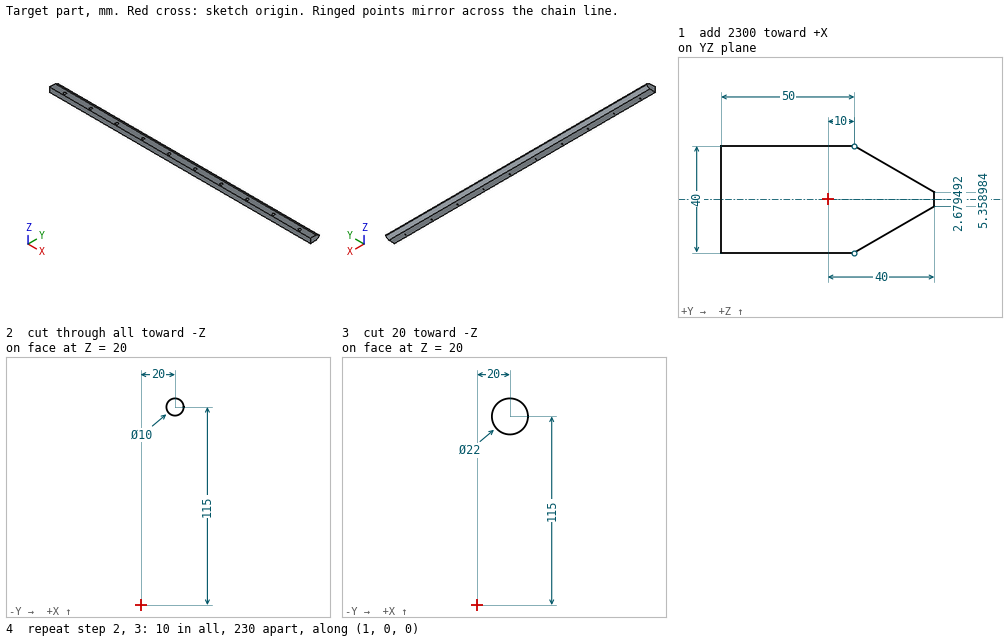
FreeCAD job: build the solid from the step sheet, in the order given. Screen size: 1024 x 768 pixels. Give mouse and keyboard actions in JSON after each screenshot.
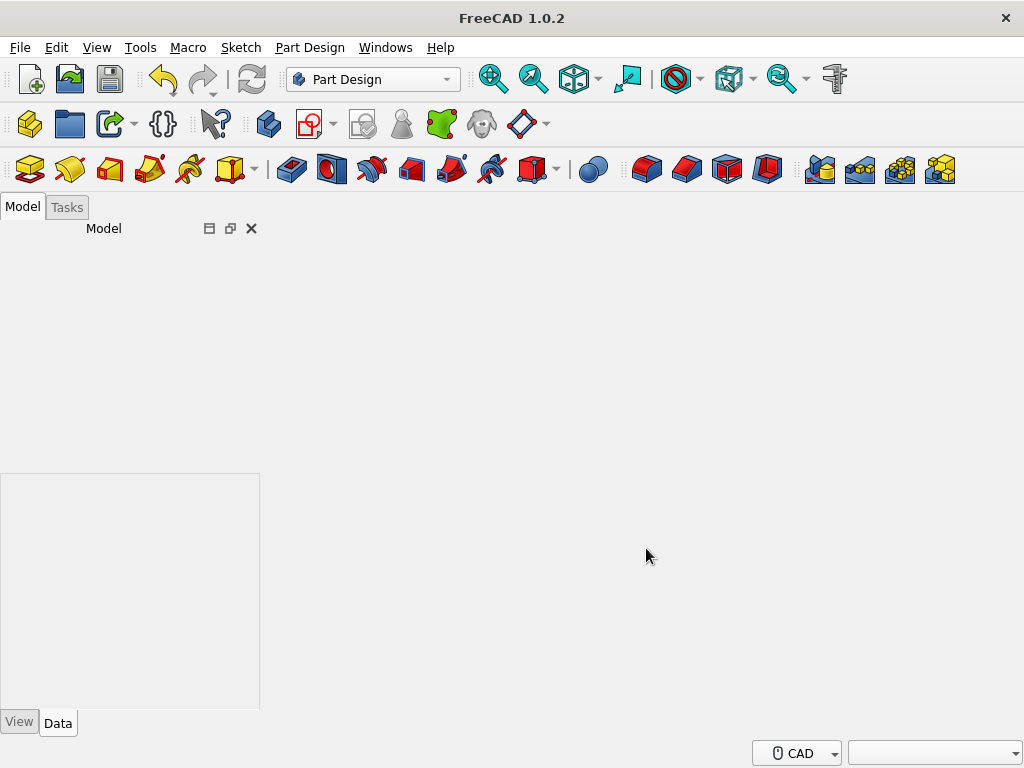
{"action": "key", "text": "ctrl+n"}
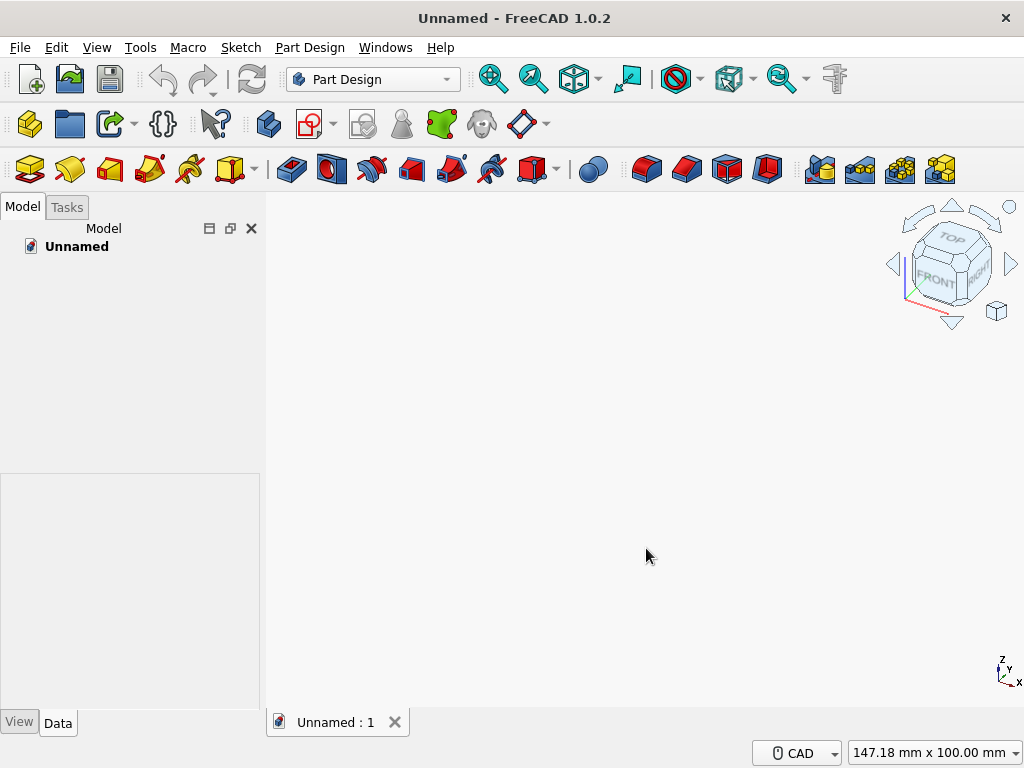
{"action": "left_click", "coordinate": [310, 124]}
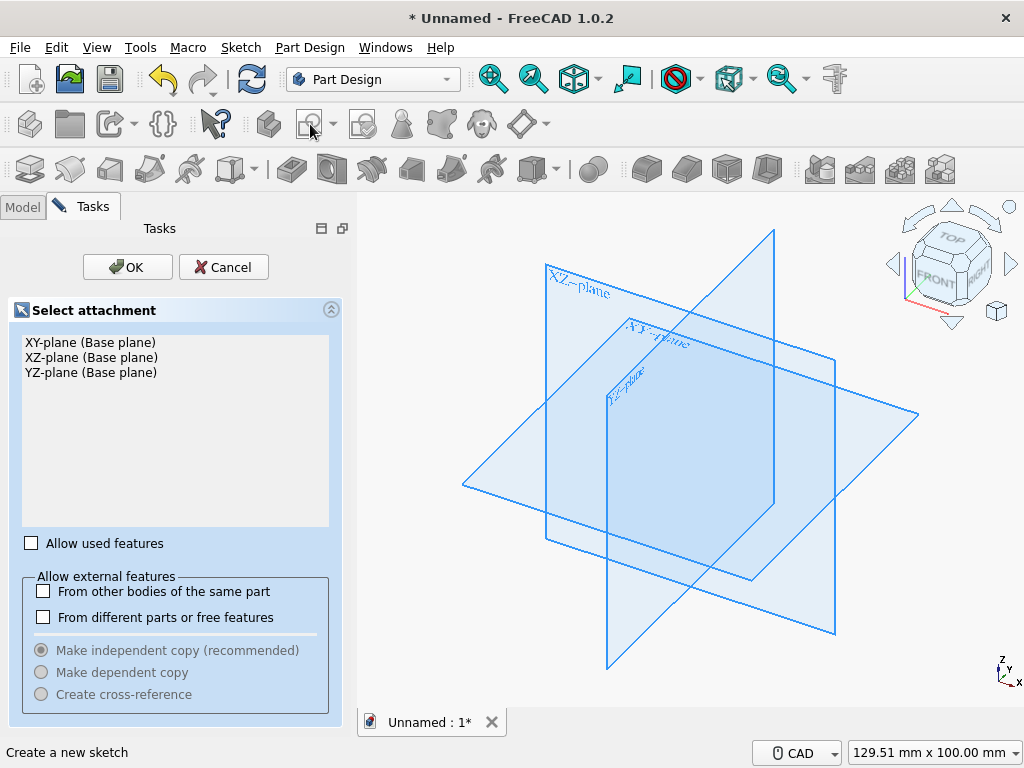
{"action": "left_click", "coordinate": [82, 372]}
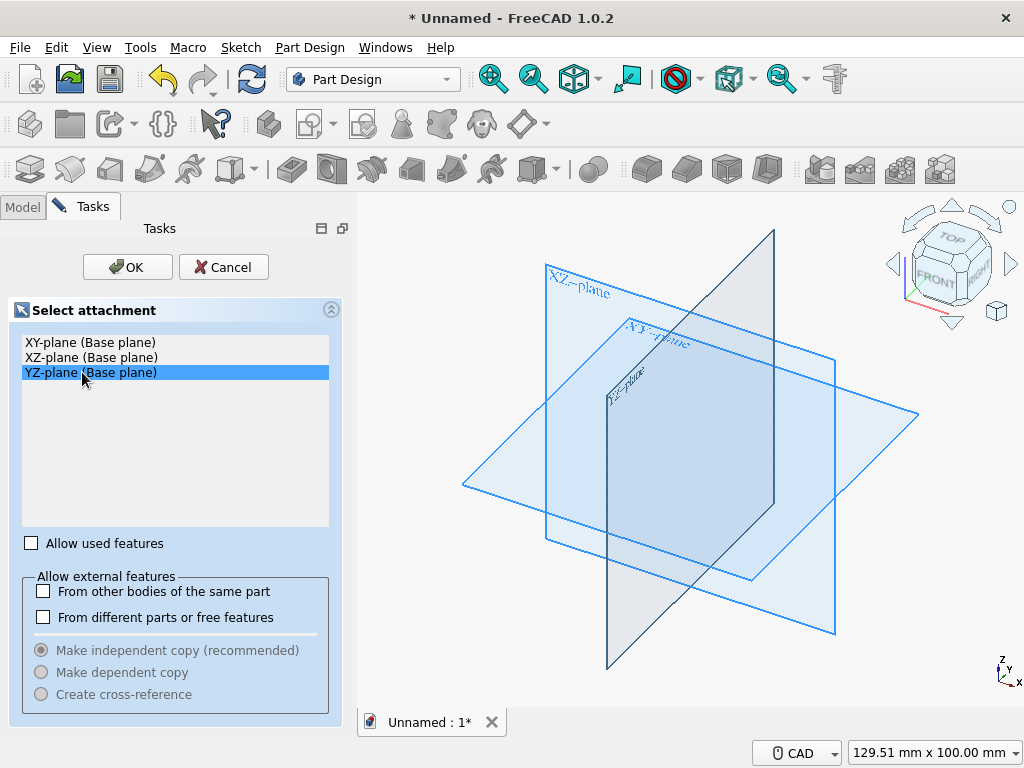
{"action": "left_click", "coordinate": [128, 267]}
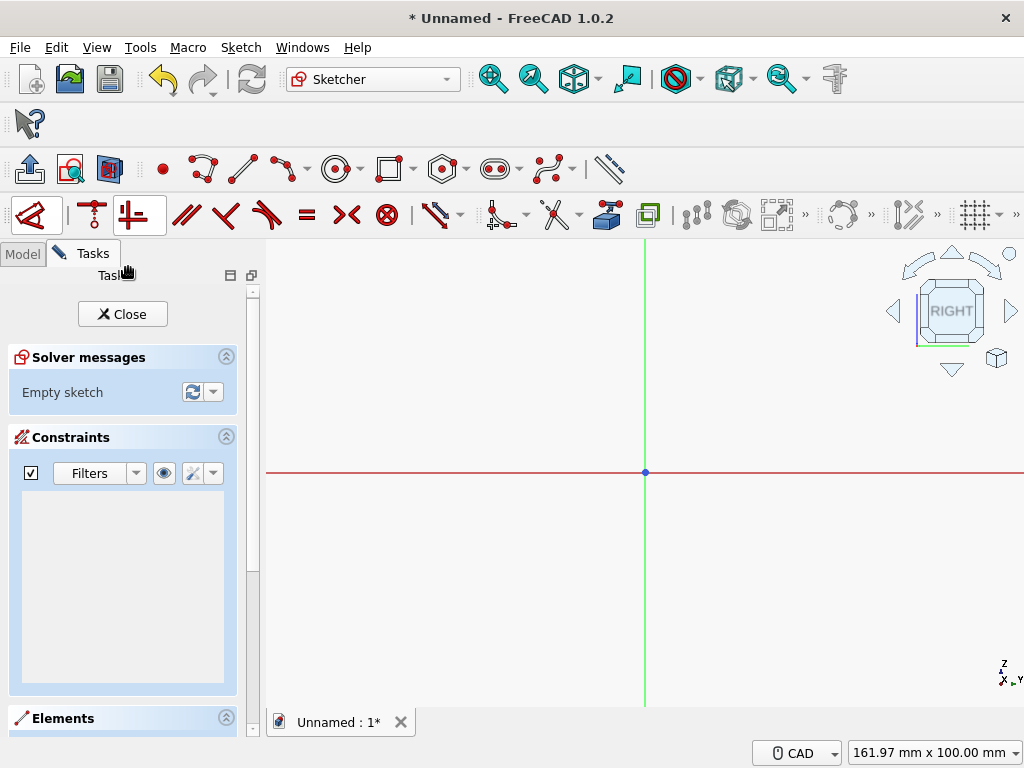
{"action": "key", "text": "g m"}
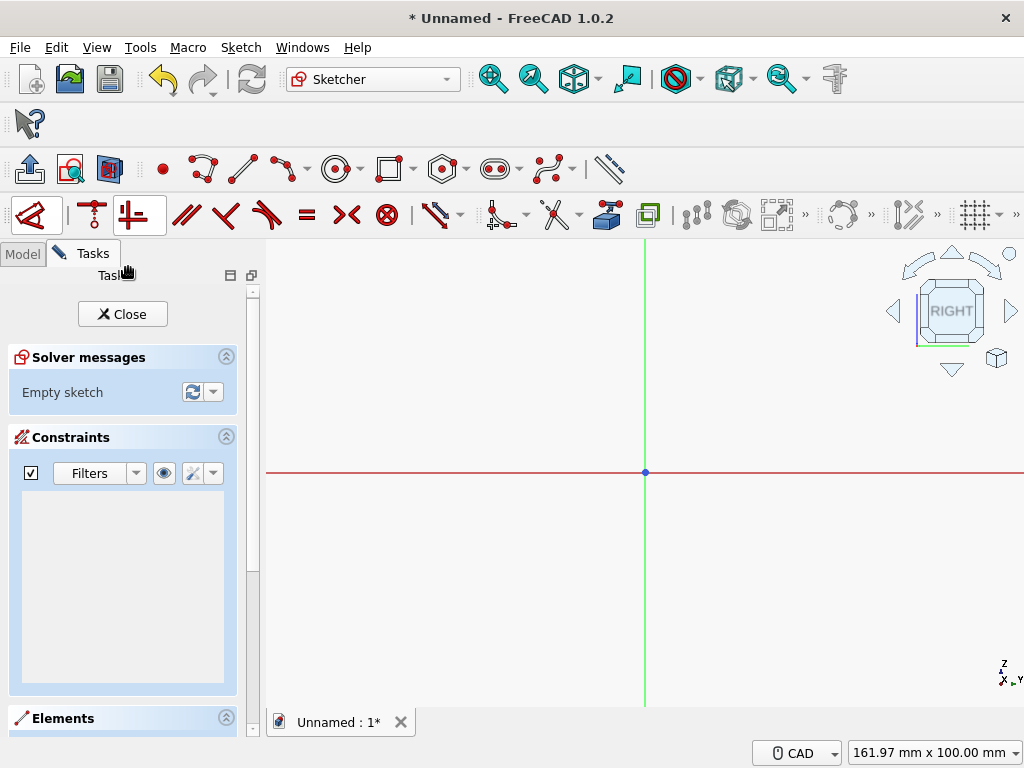
{"action": "left_click", "coordinate": [692, 379]}
{"action": "left_click", "coordinate": [458, 379]}
{"action": "left_click", "coordinate": [458, 567]}
{"action": "left_click", "coordinate": [692, 567]}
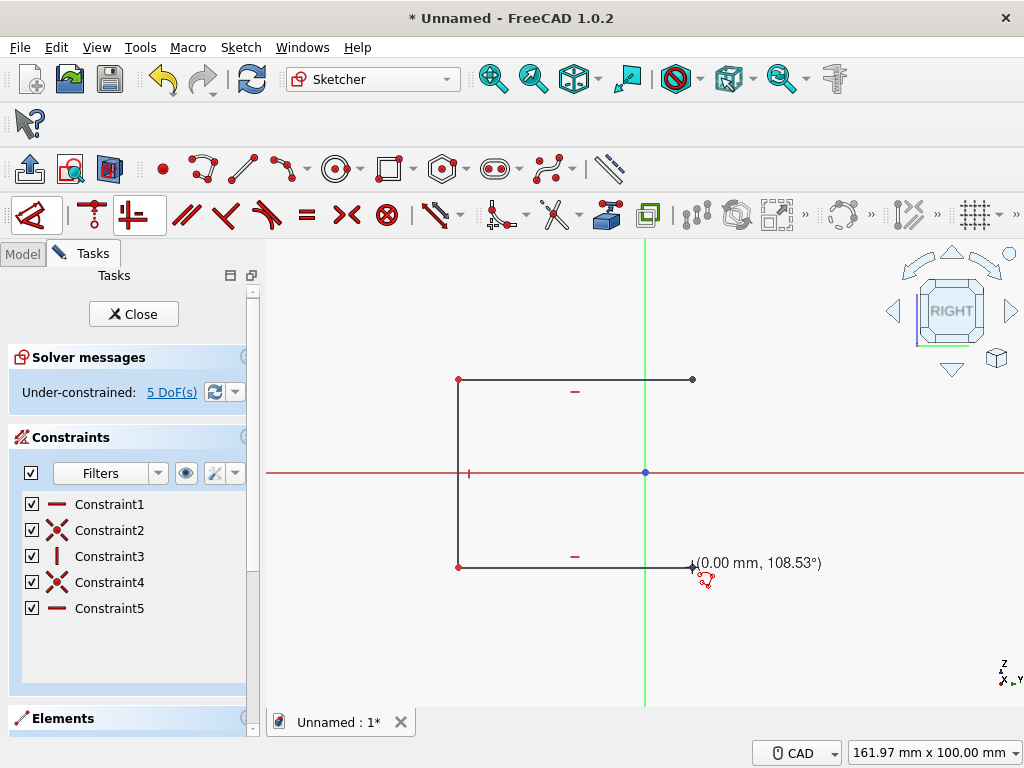
{"action": "scroll", "coordinate": [832, 486], "scroll_direction": "up", "scroll_amount": 2}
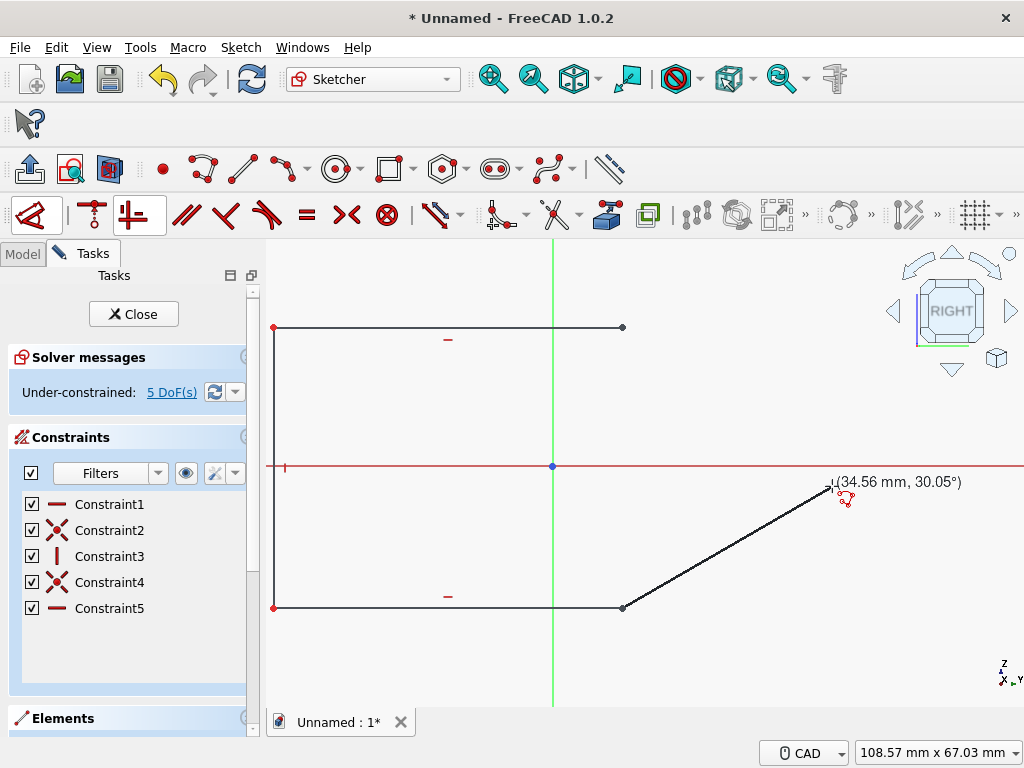
{"action": "left_click", "coordinate": [832, 485]}
{"action": "left_click", "coordinate": [832, 448]}
{"action": "left_click", "coordinate": [623, 328]}
{"action": "key", "text": "Escape"}
{"action": "key", "text": "Escape"}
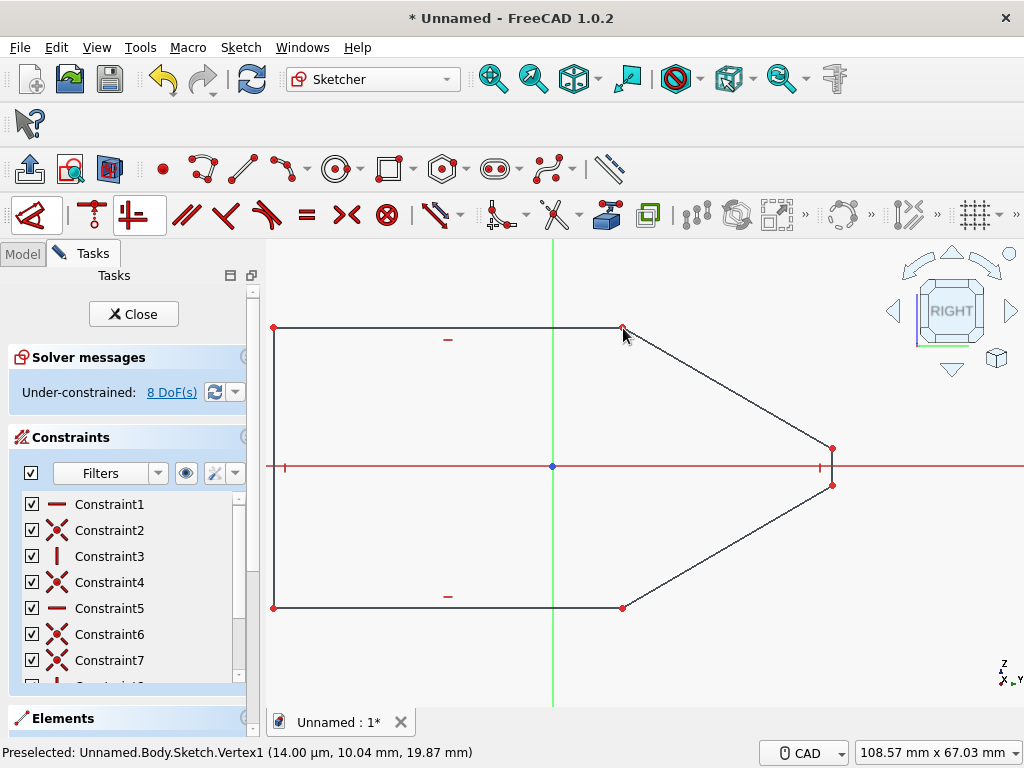
{"action": "left_click", "coordinate": [623, 328]}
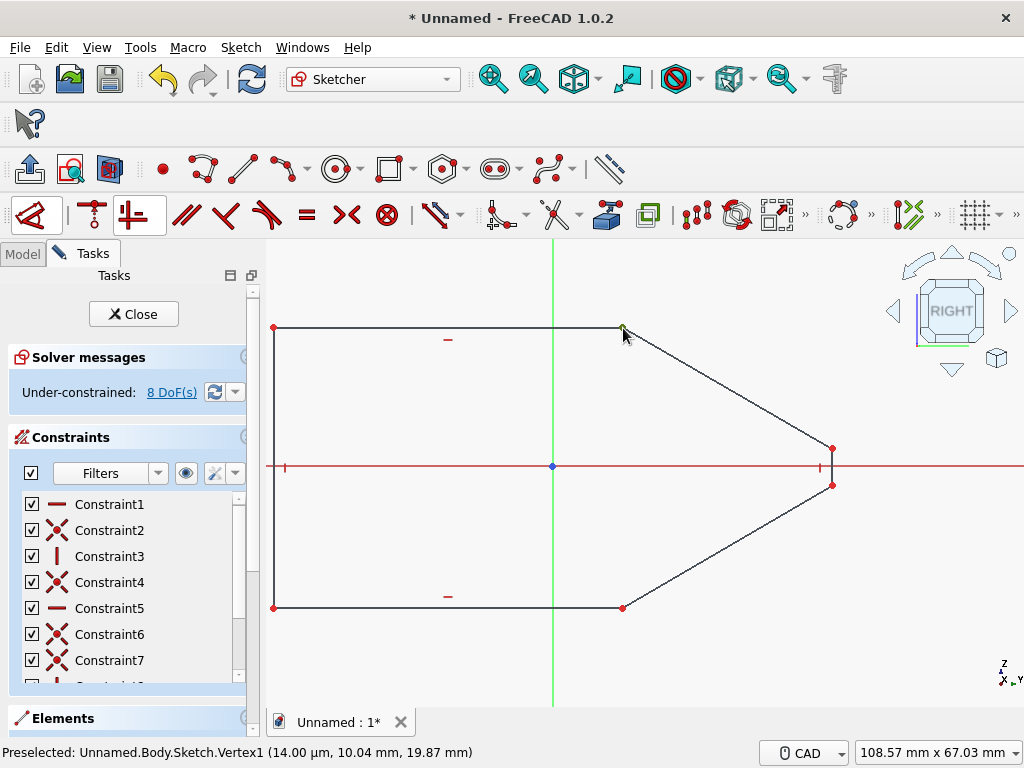
{"action": "left_click", "coordinate": [623, 608]}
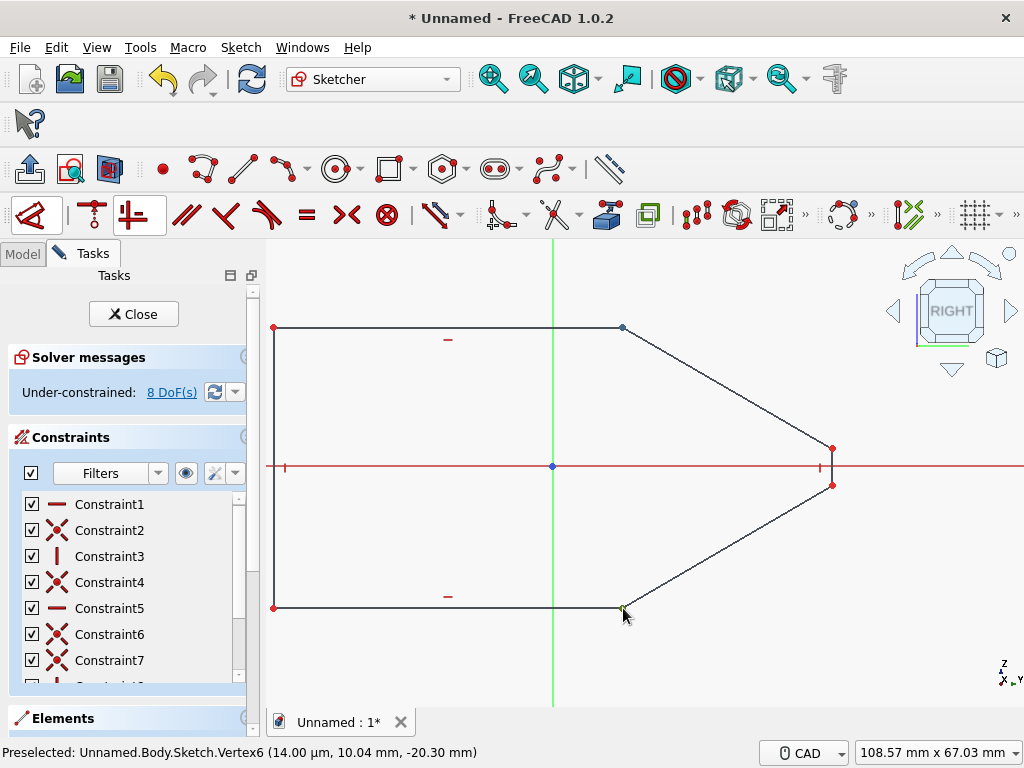
{"action": "left_click", "coordinate": [334, 466]}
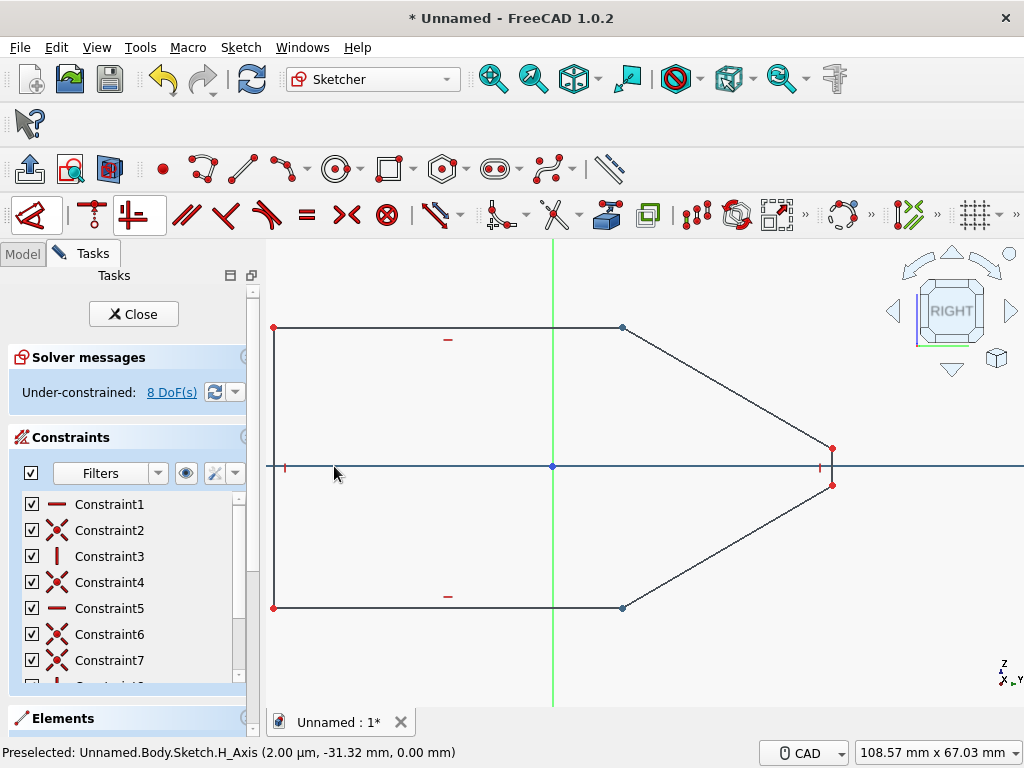
{"action": "key", "text": "s"}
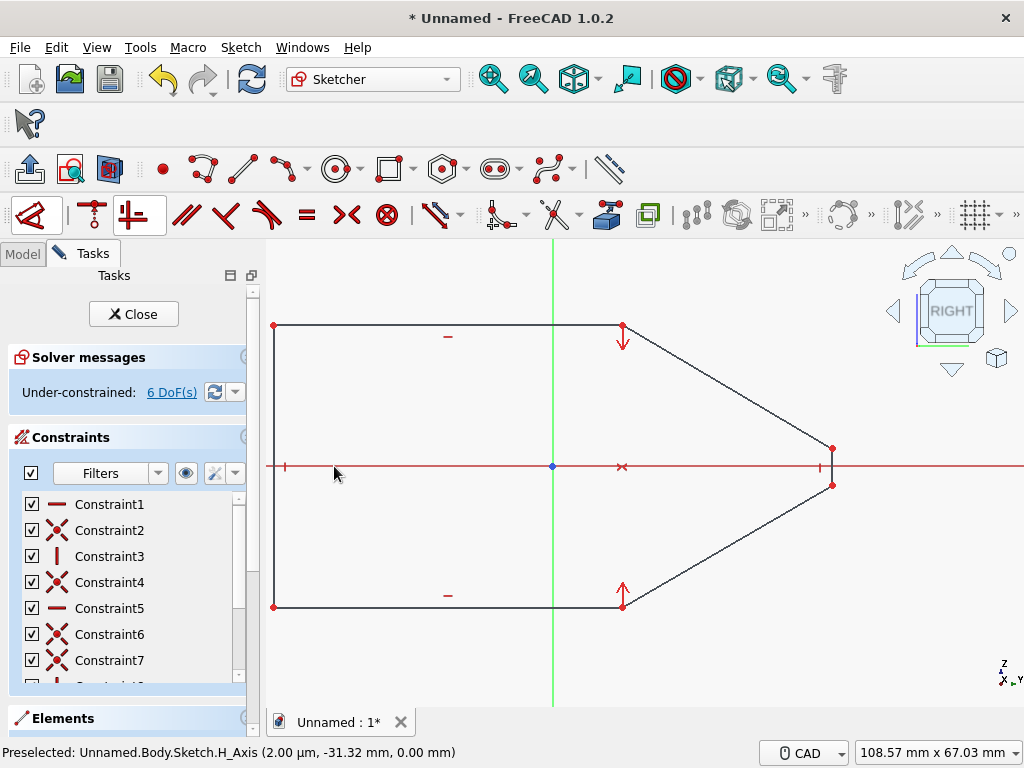
{"action": "left_click", "coordinate": [518, 325]}